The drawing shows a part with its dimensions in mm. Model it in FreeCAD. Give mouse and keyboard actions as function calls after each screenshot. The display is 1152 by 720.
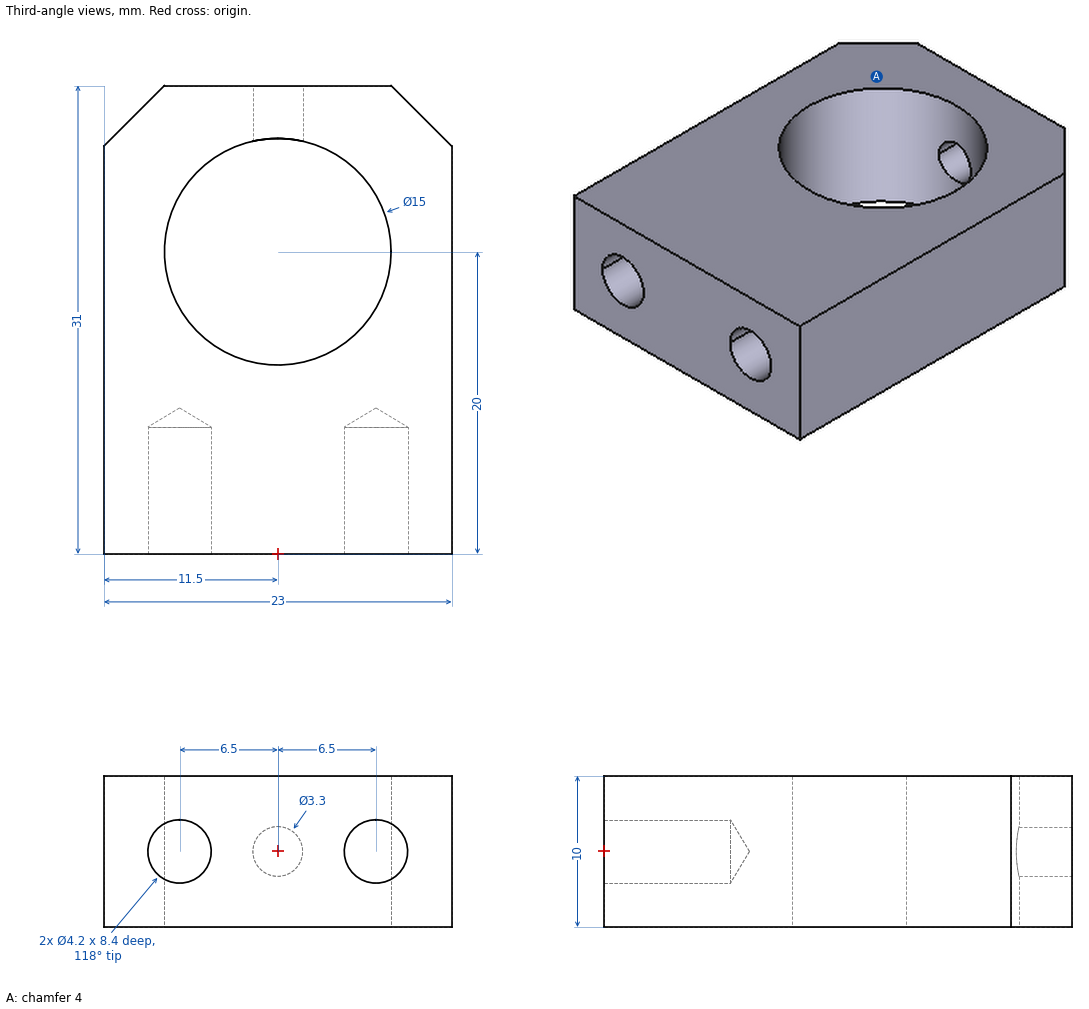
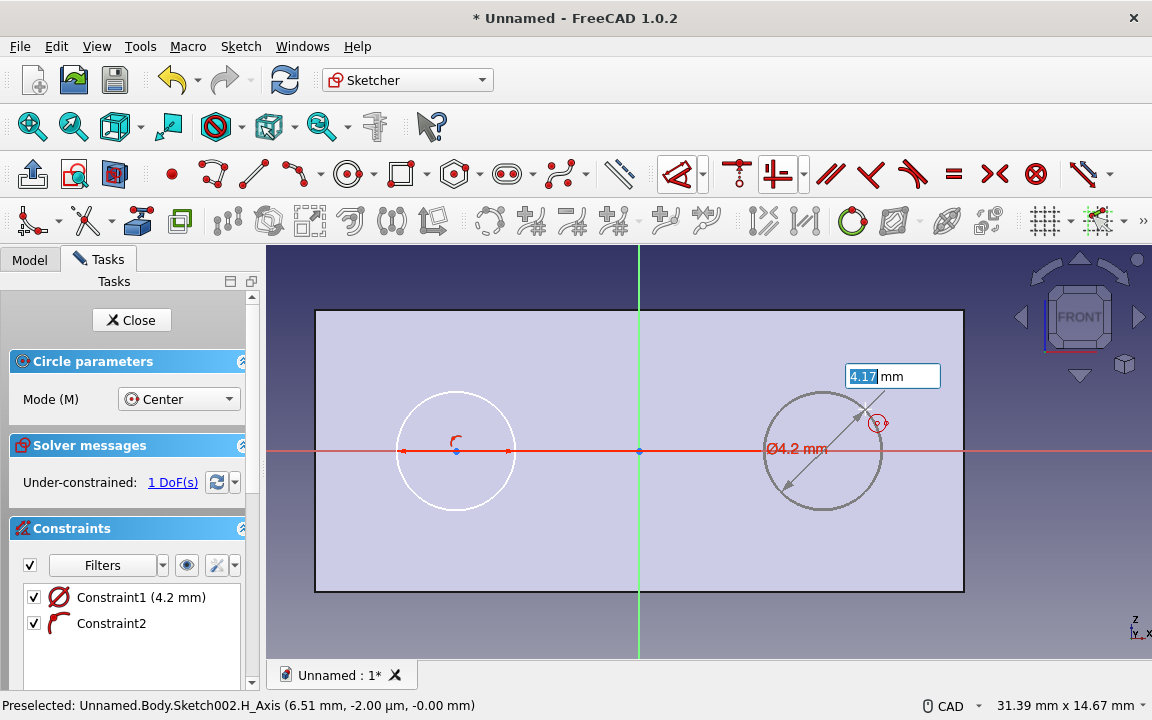
text(4.2)
key(Return)
key(Escape)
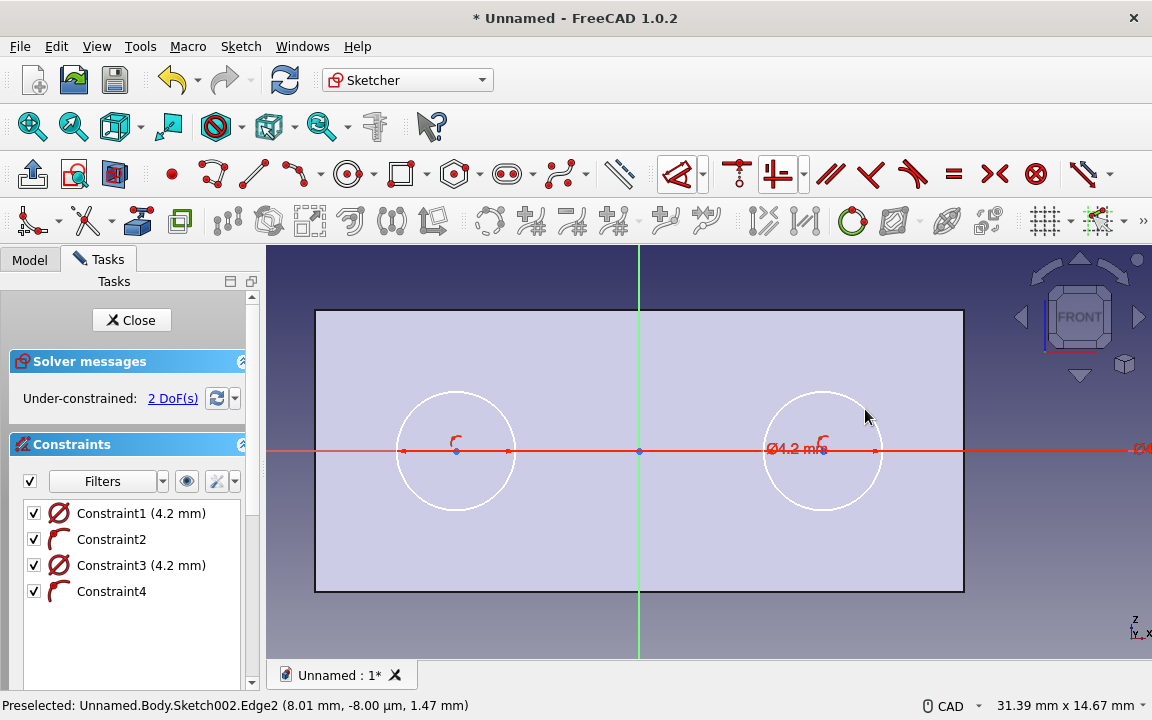
click(676, 174)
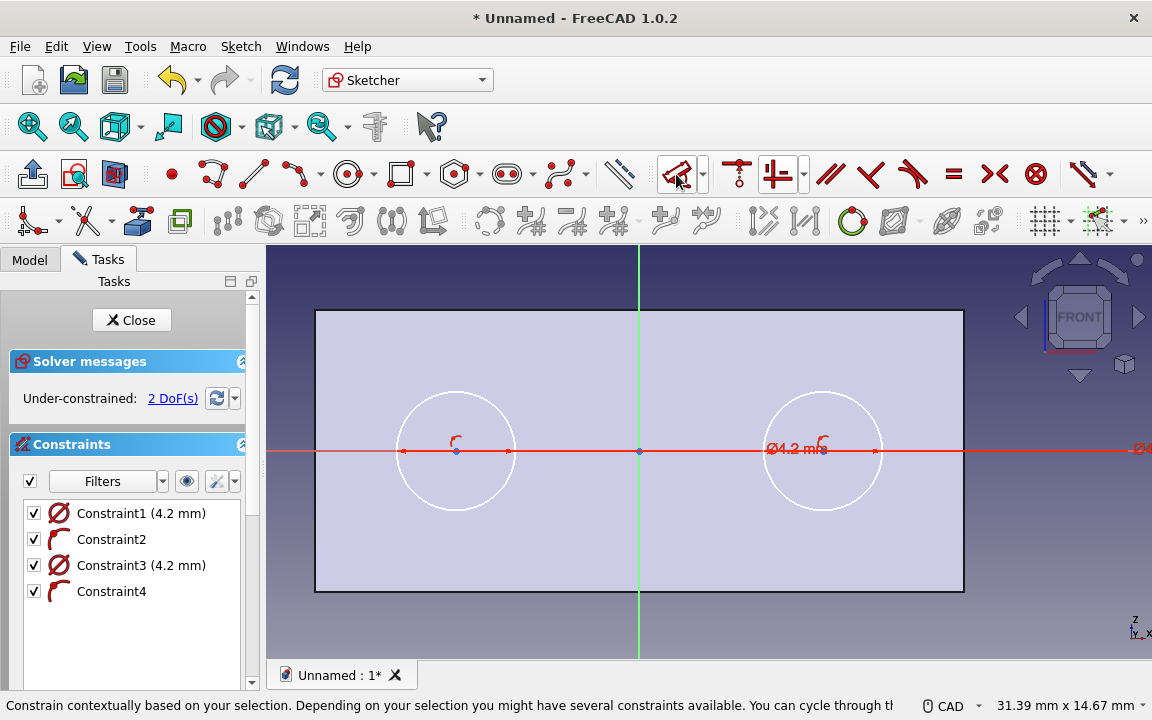
click(456, 451)
click(548, 485)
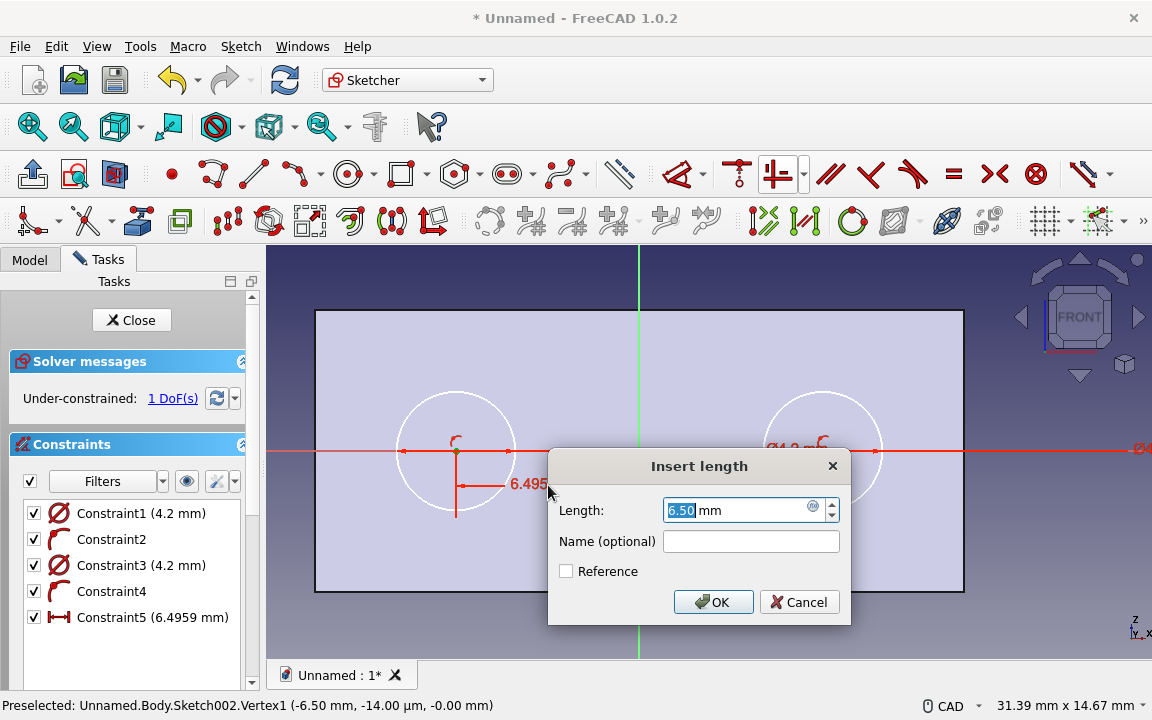
text(6.5)
key(Return)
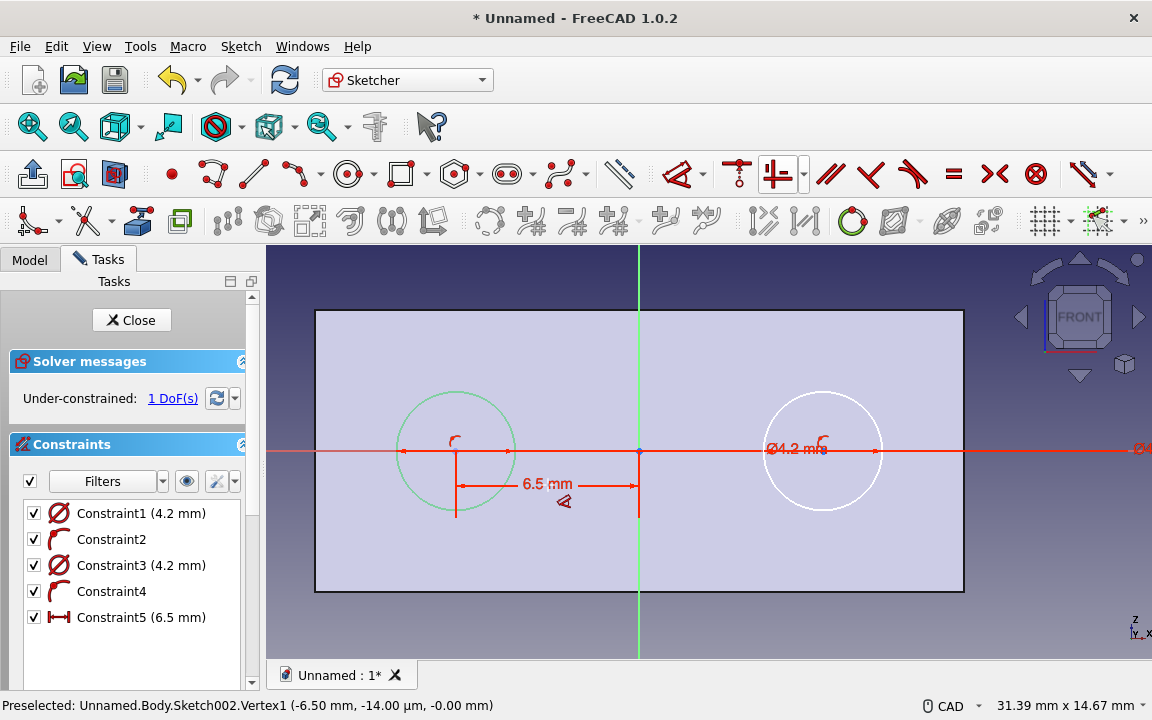
click(823, 451)
click(731, 485)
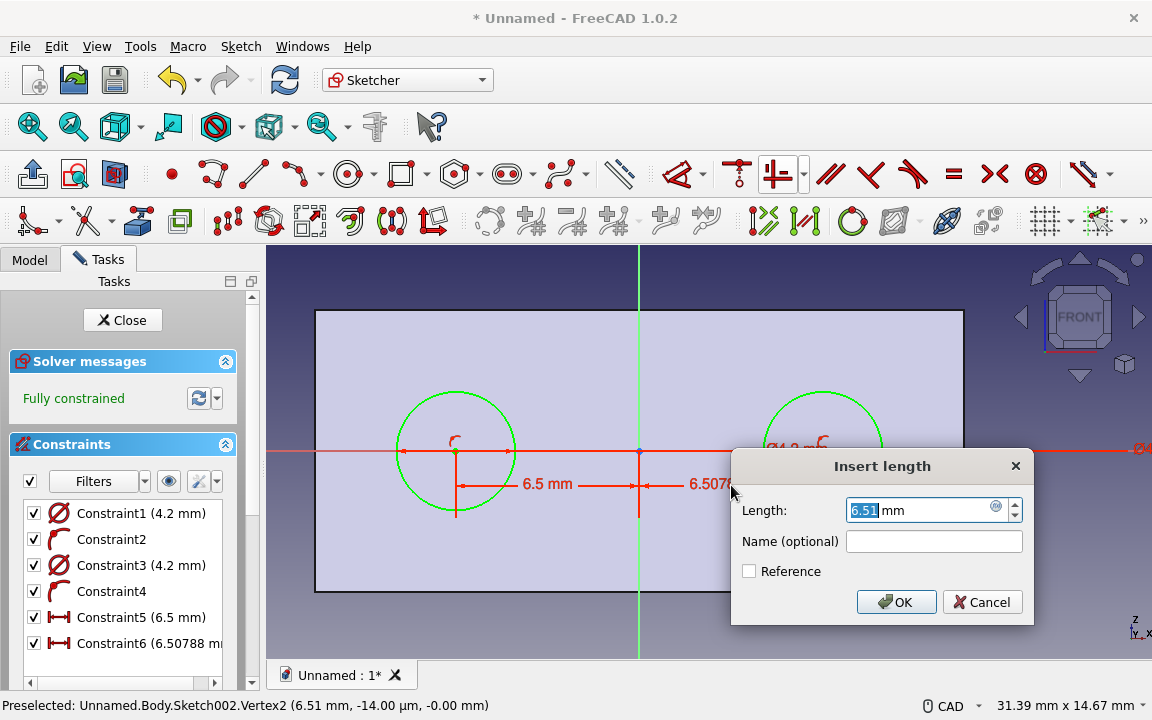
text(6.5)
key(Return)
key(Escape)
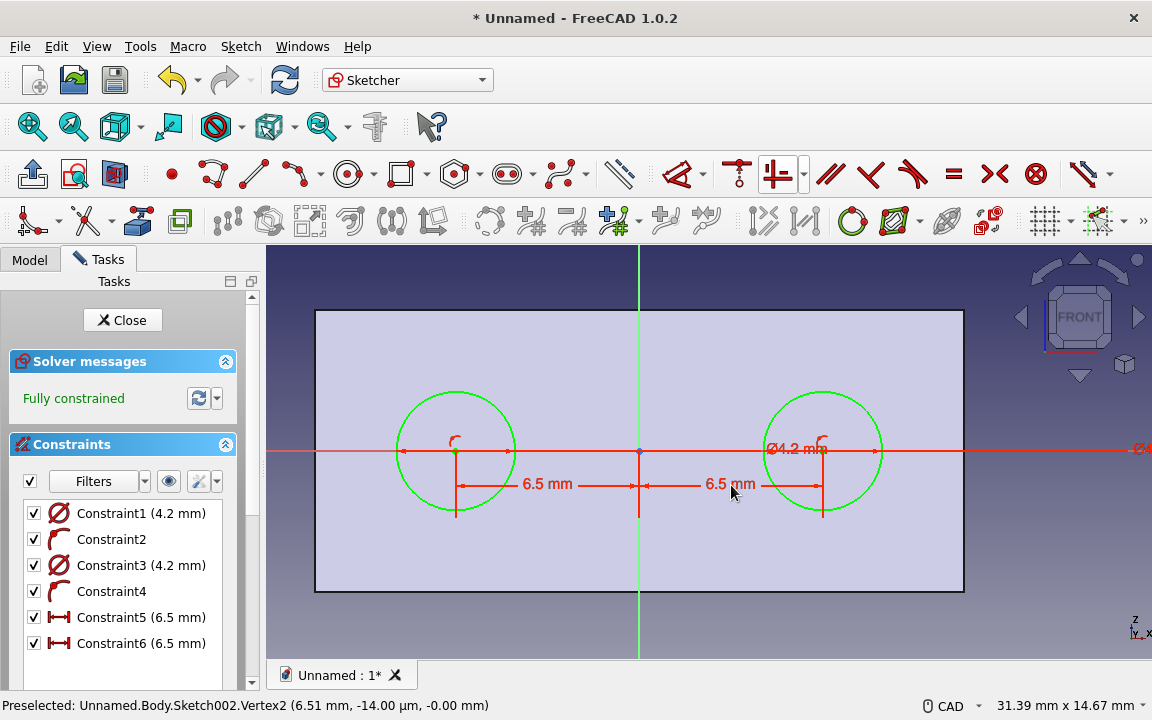
click(123, 320)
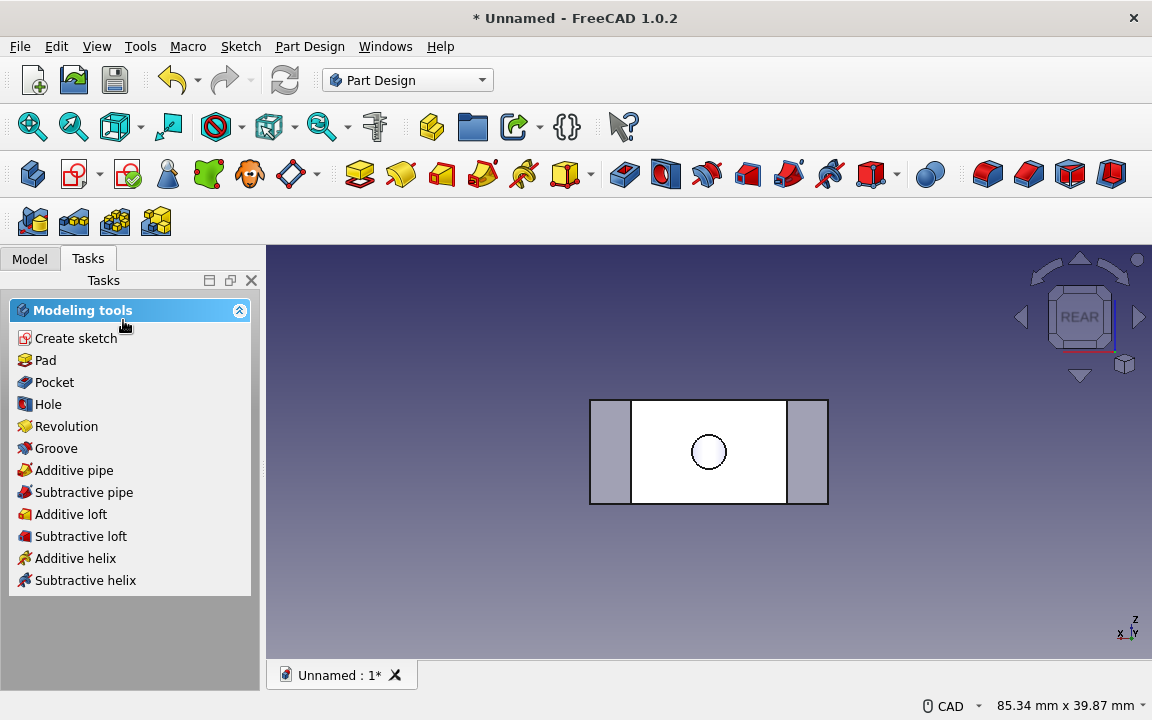
click(666, 174)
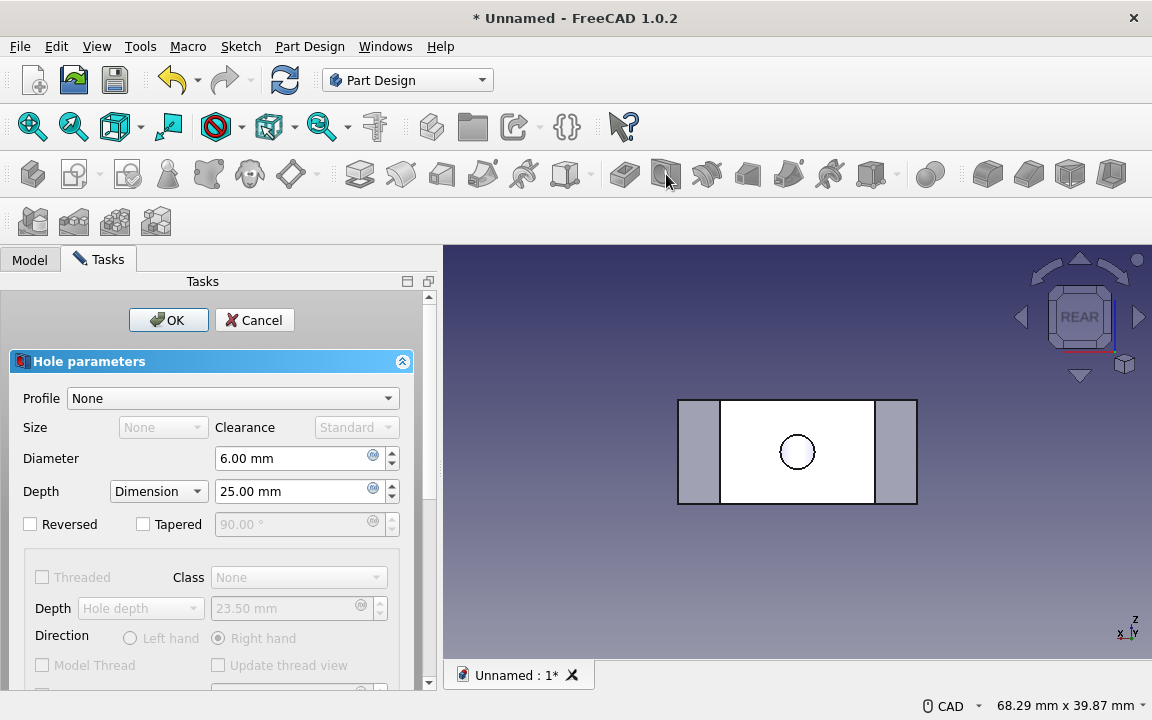
triple_click(300, 458)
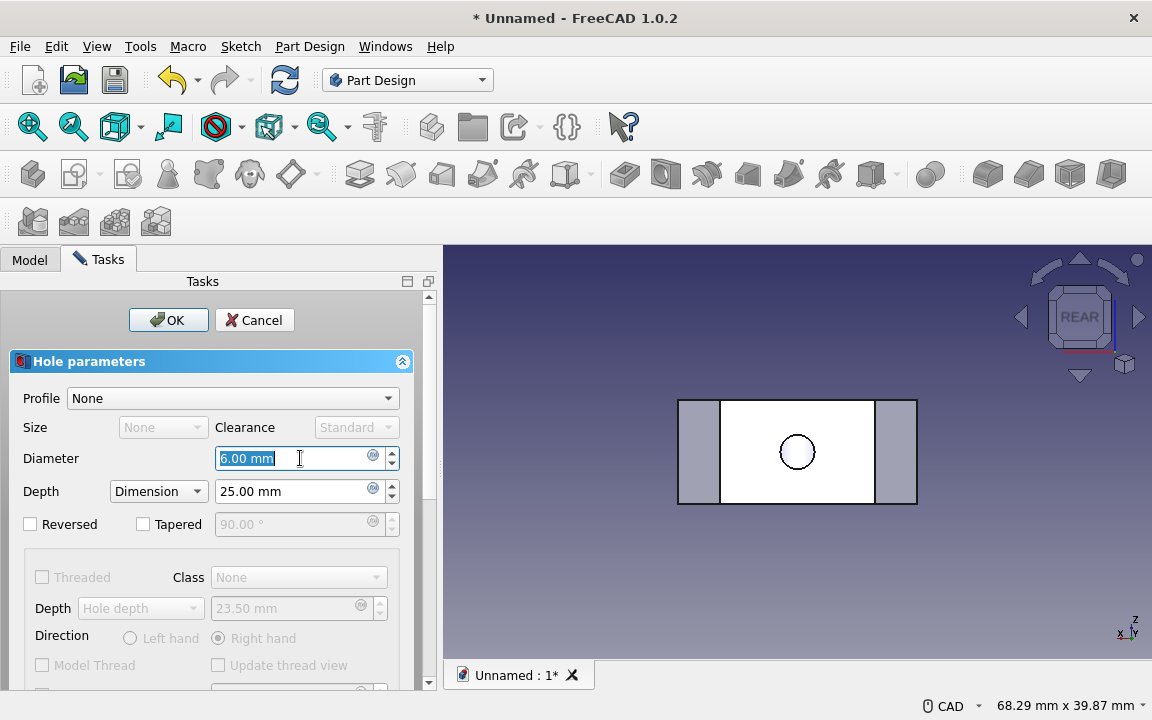
text(4.2)
key(Tab)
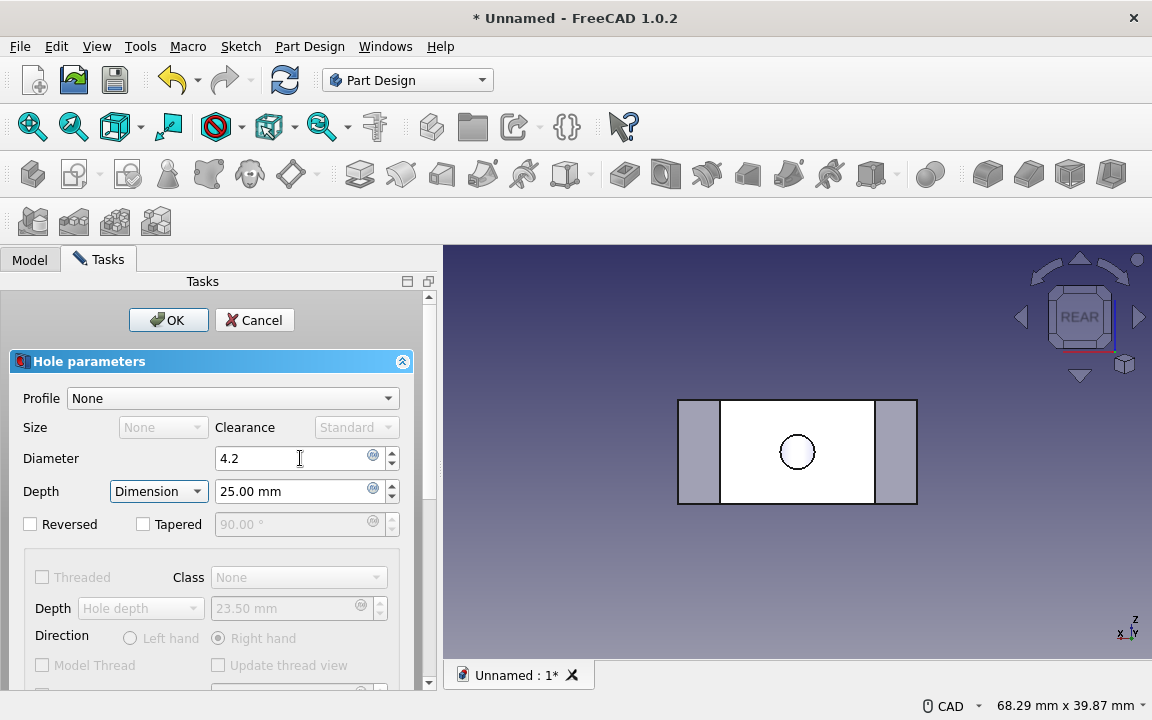
triple_click(300, 492)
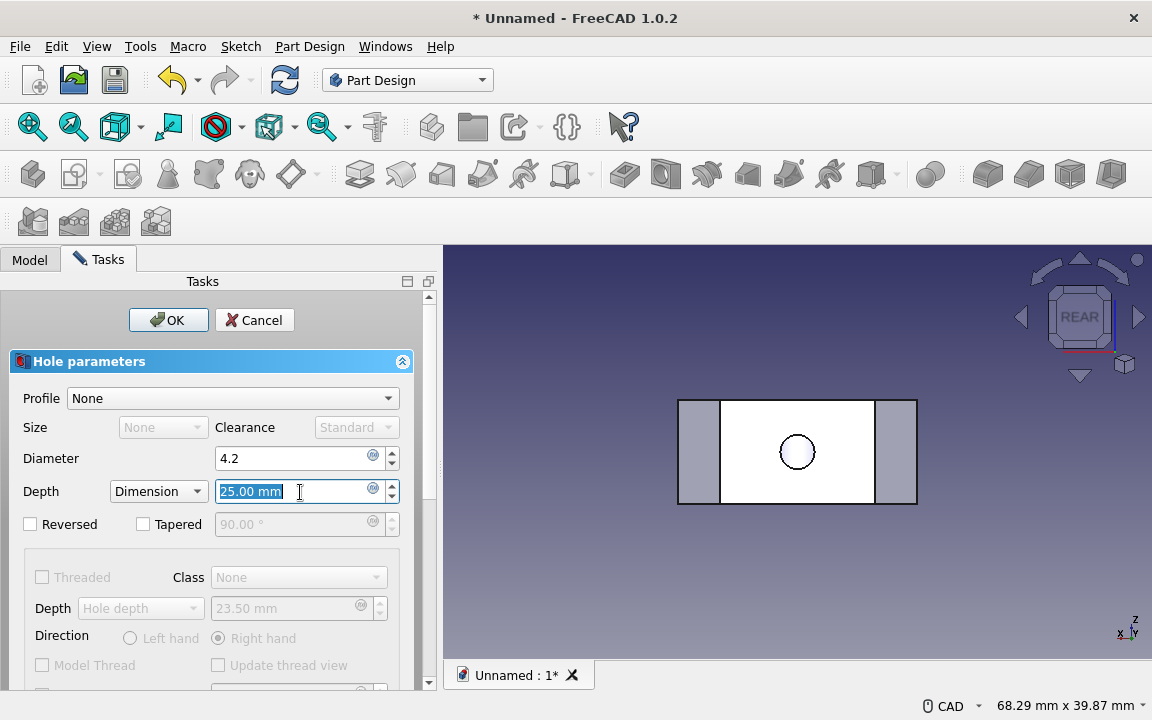
text(8.4)
key(Tab)